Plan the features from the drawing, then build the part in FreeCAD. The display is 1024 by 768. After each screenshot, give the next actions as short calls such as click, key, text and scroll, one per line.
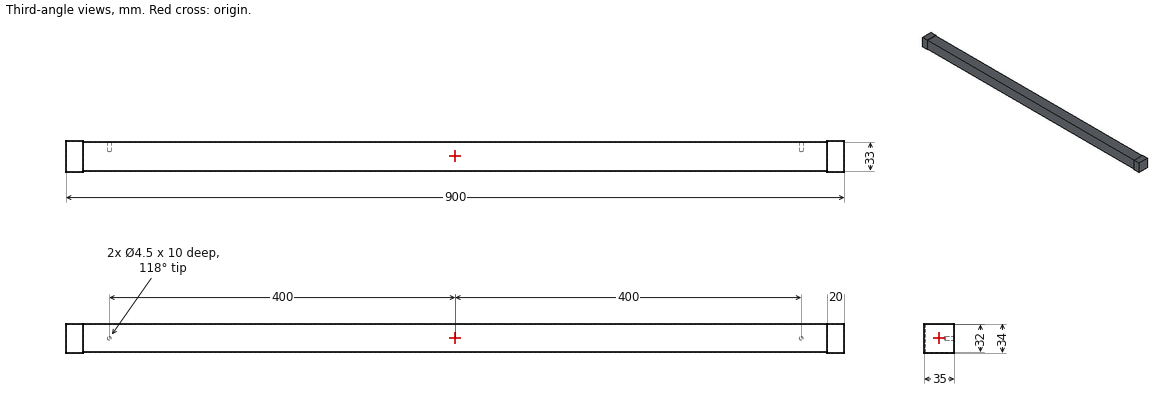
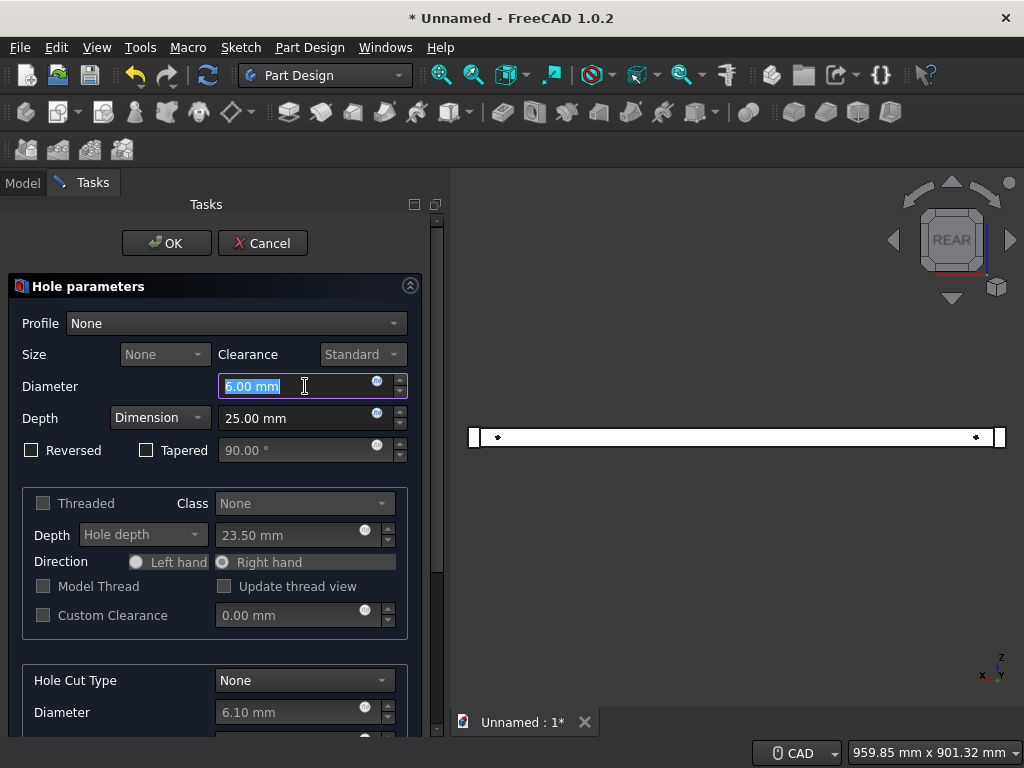
text(4.5)
key(Tab)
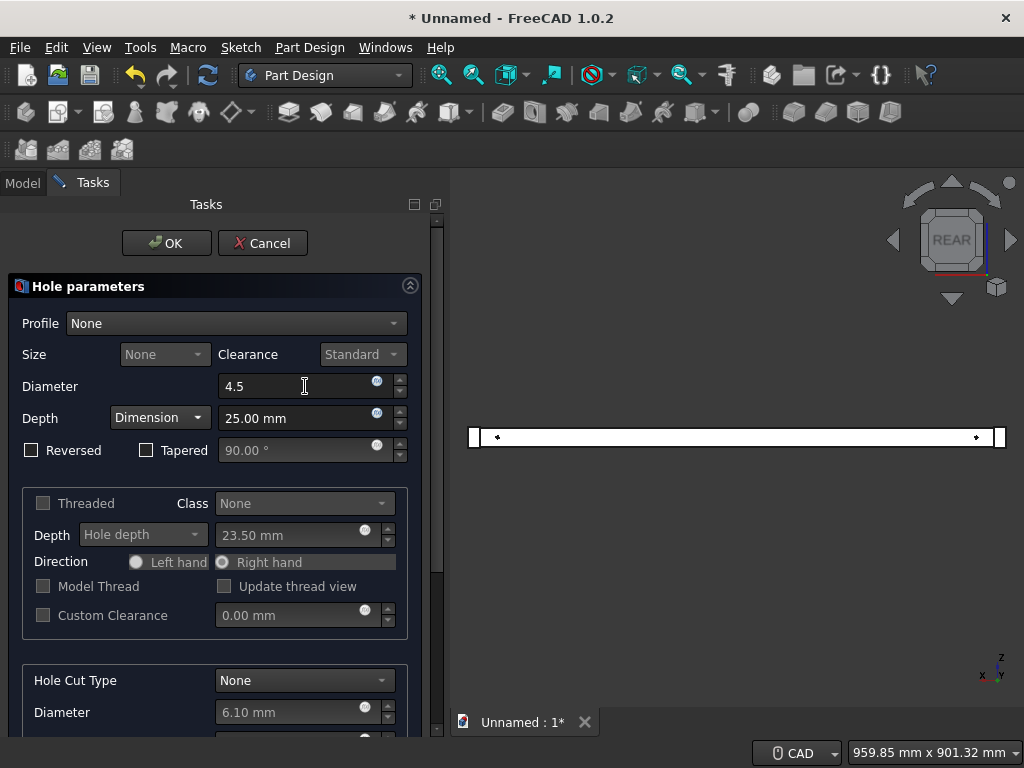
triple_click(305, 418)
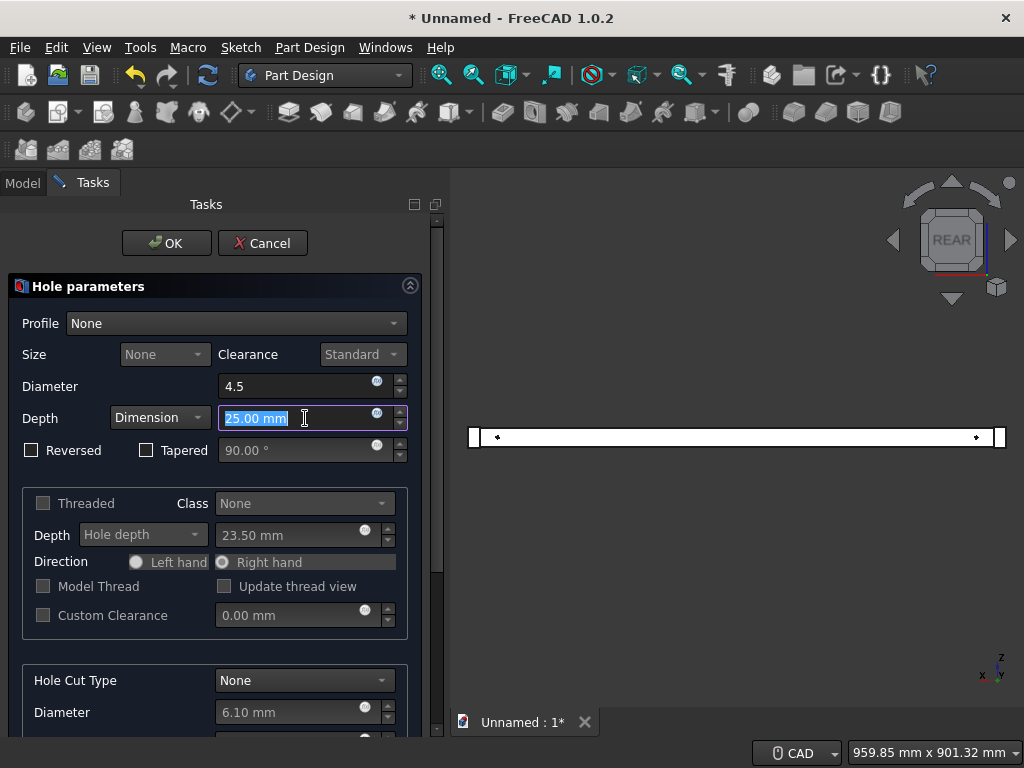
text(10)
key(Tab)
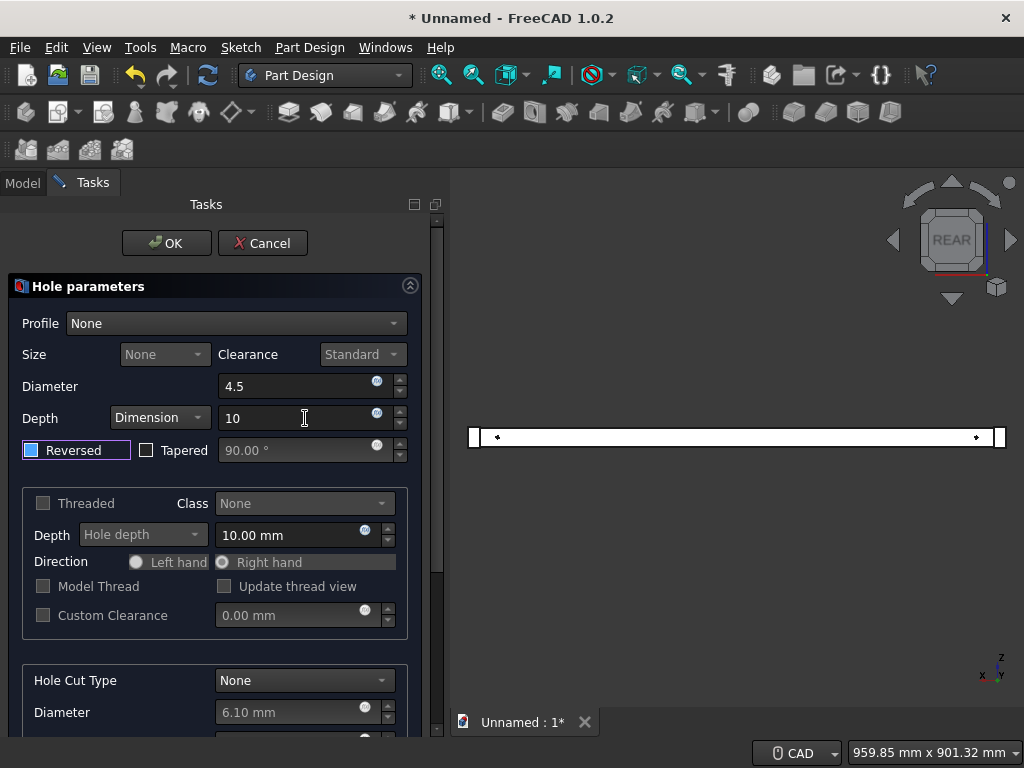
click(167, 243)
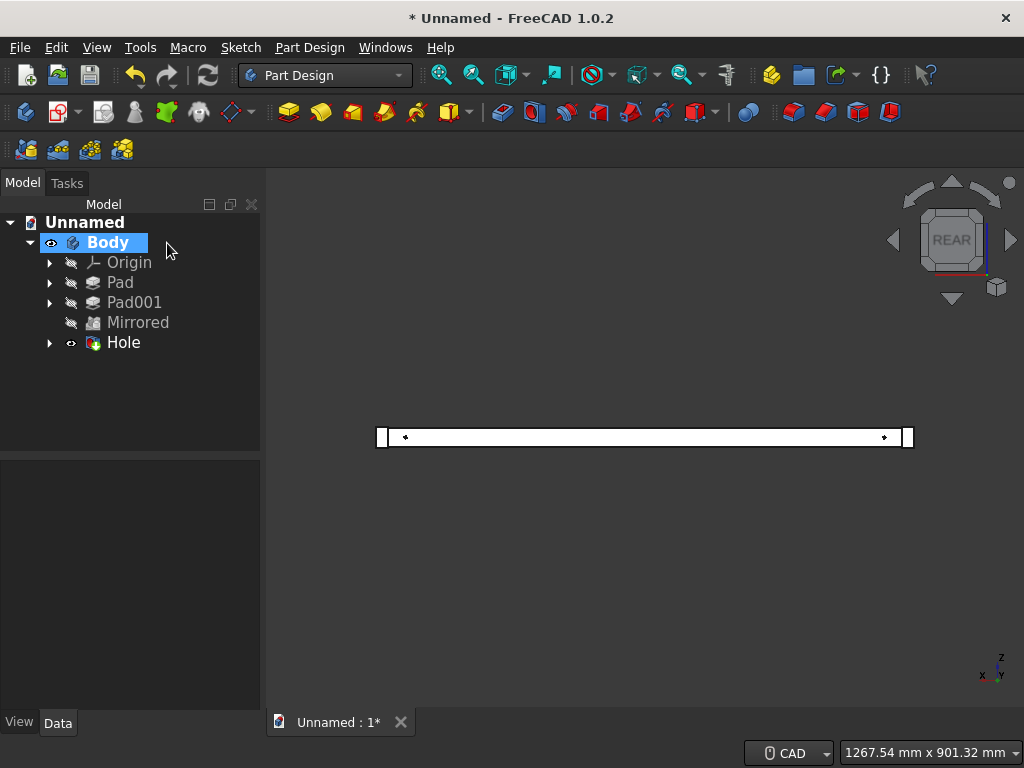
key(0)